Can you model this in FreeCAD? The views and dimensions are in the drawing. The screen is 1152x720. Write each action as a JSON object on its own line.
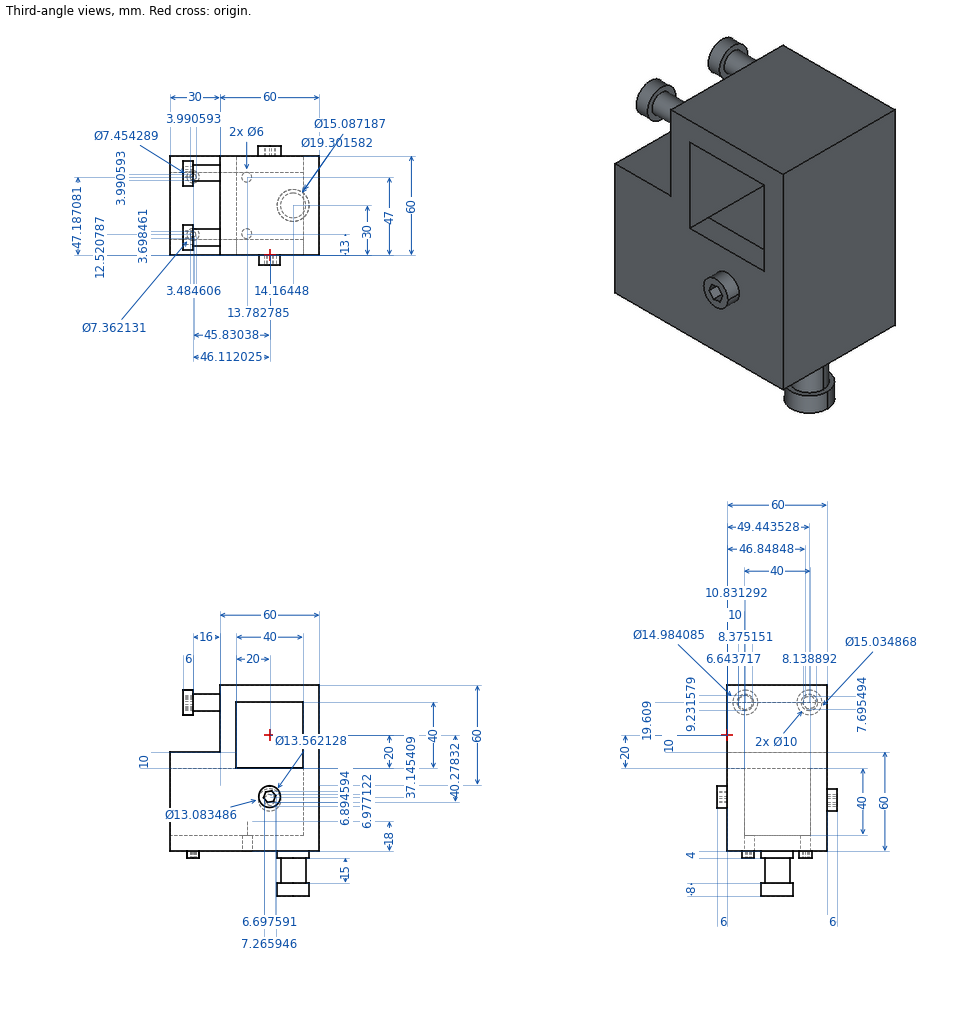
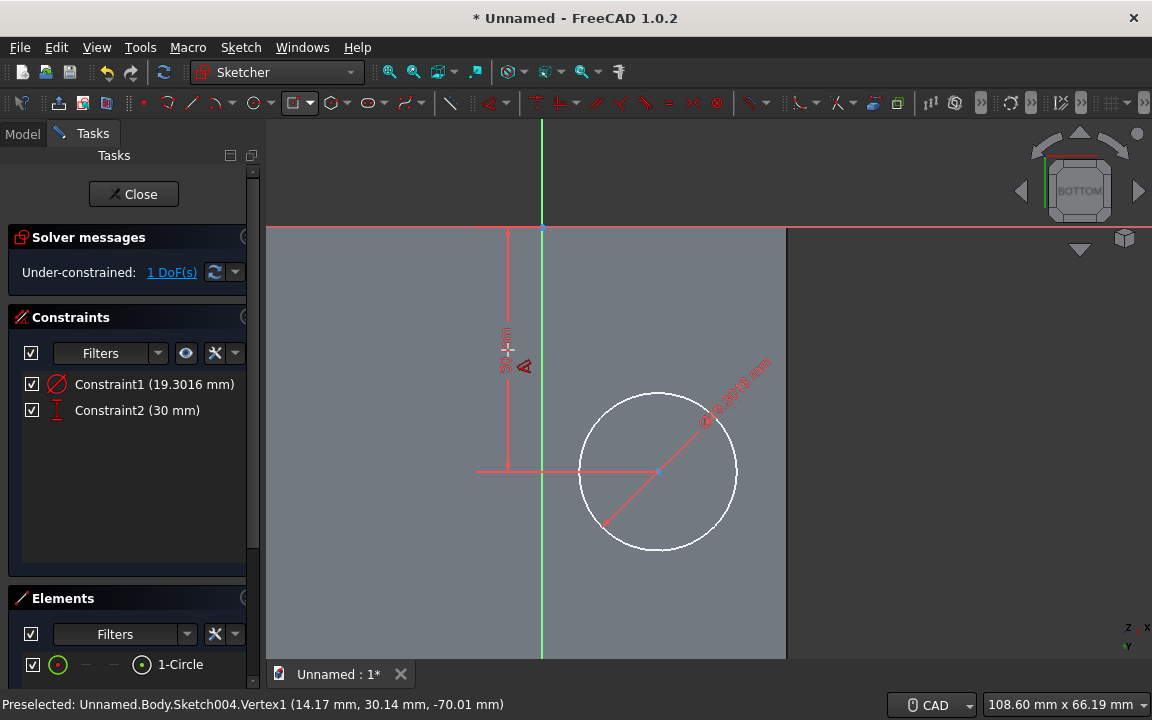
{"action": "left_click", "coordinate": [658, 472]}
{"action": "left_click", "coordinate": [600, 193]}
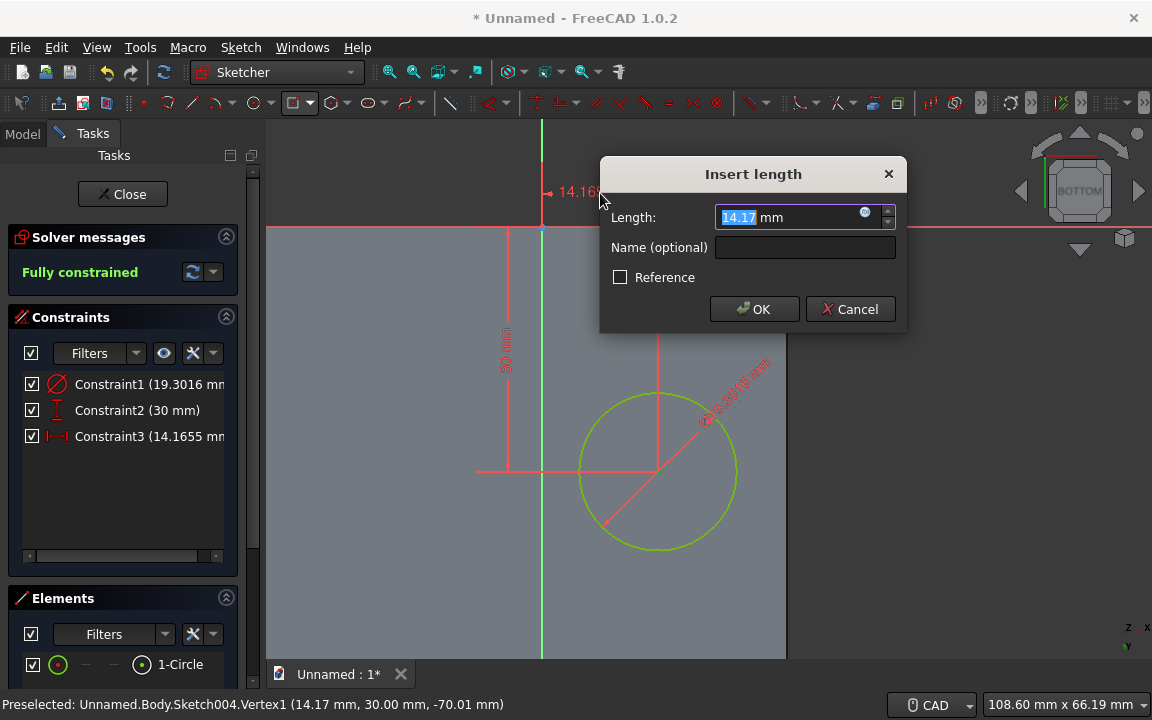
{"action": "type", "text": "14.16448"}
{"action": "key", "text": "Return"}
{"action": "key", "text": "Escape"}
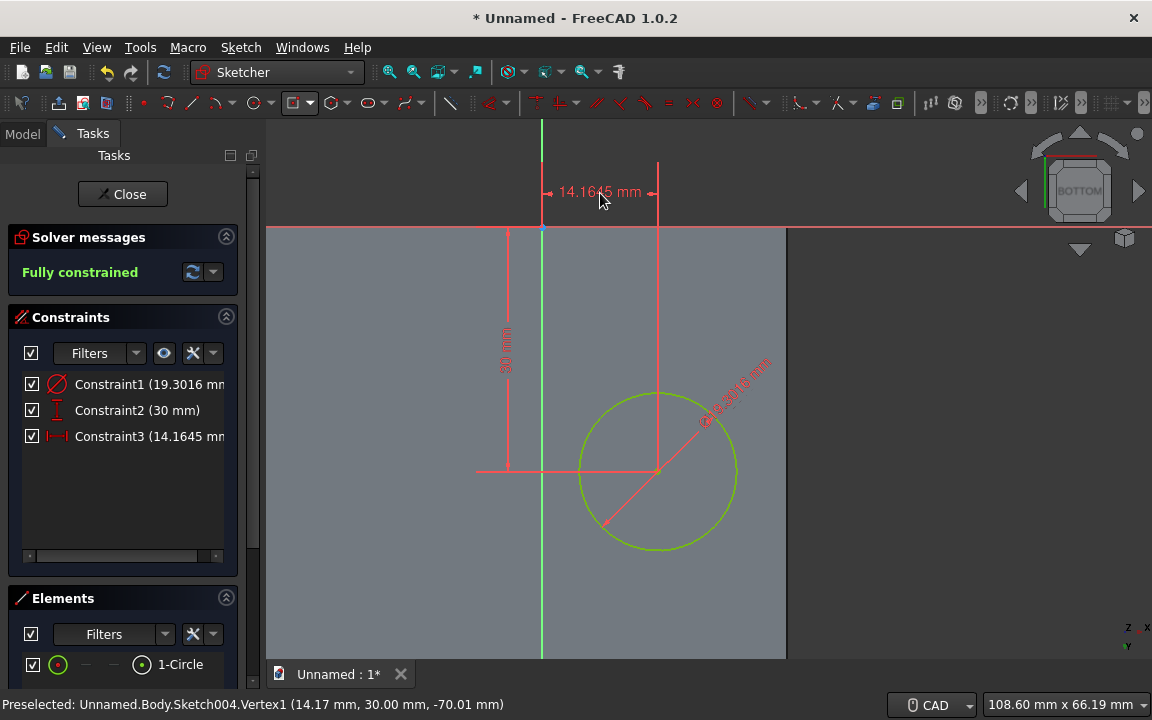
{"action": "left_click", "coordinate": [123, 194]}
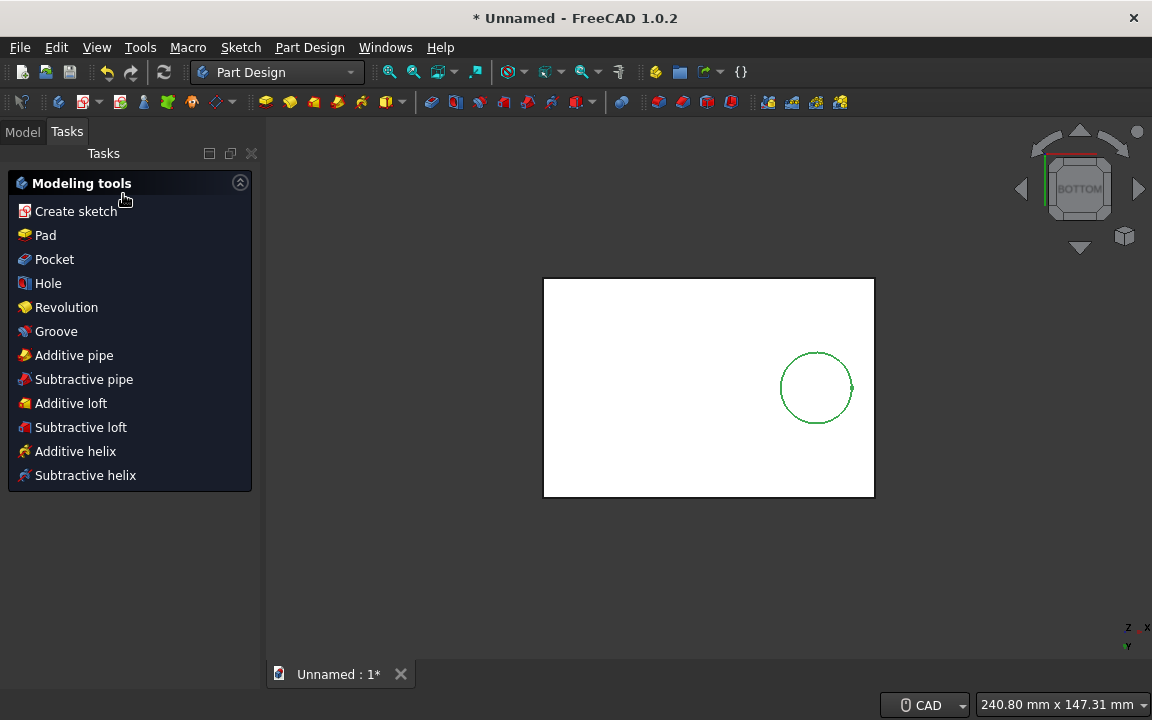
{"action": "left_click", "coordinate": [266, 102]}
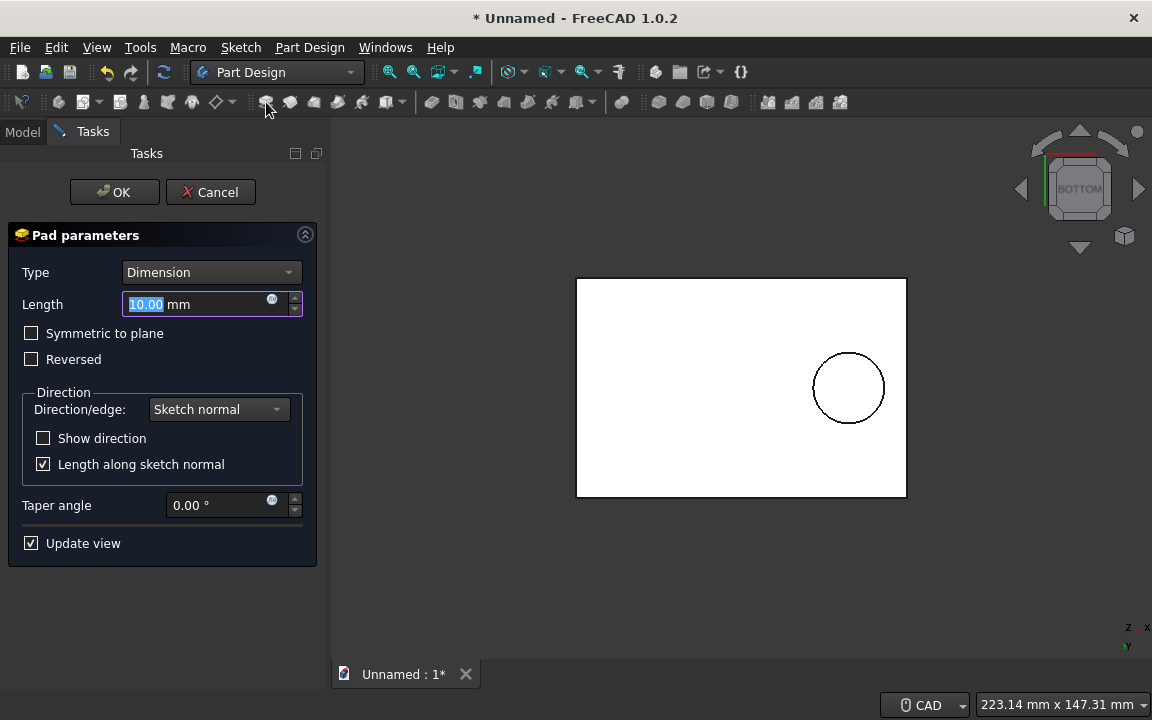
{"action": "type", "text": "4"}
{"action": "key", "text": "Tab"}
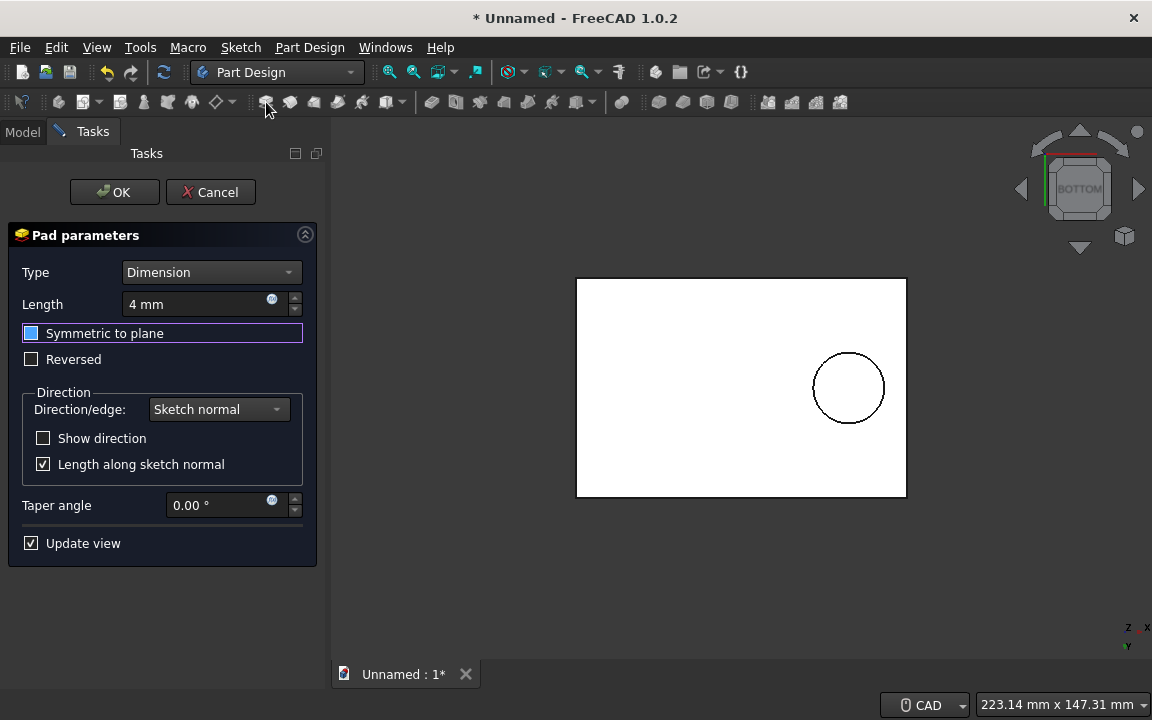
{"action": "left_click", "coordinate": [115, 192]}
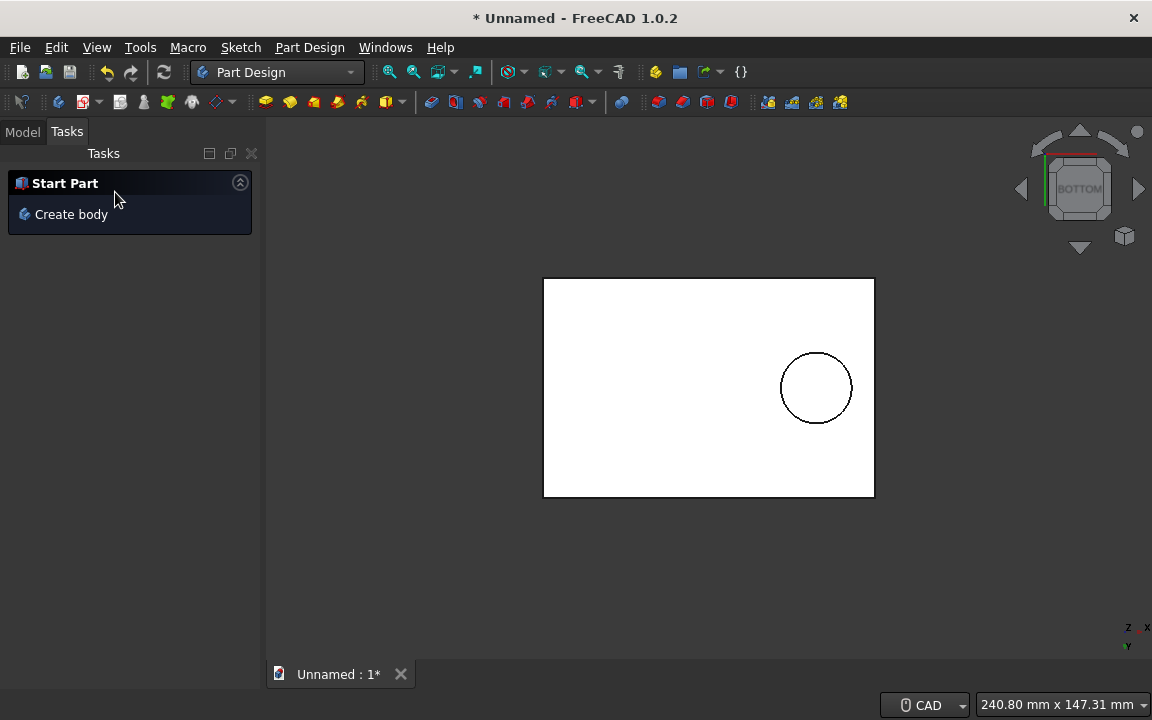
{"action": "left_click", "coordinate": [390, 72]}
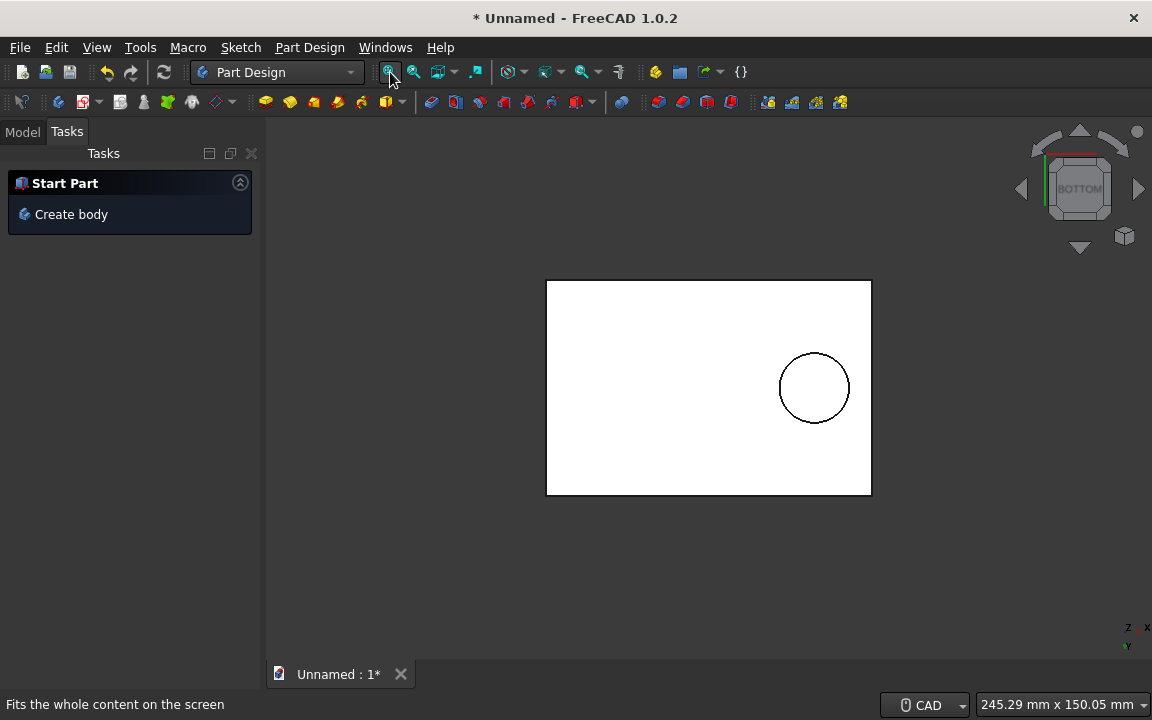
{"action": "left_click", "coordinate": [814, 387]}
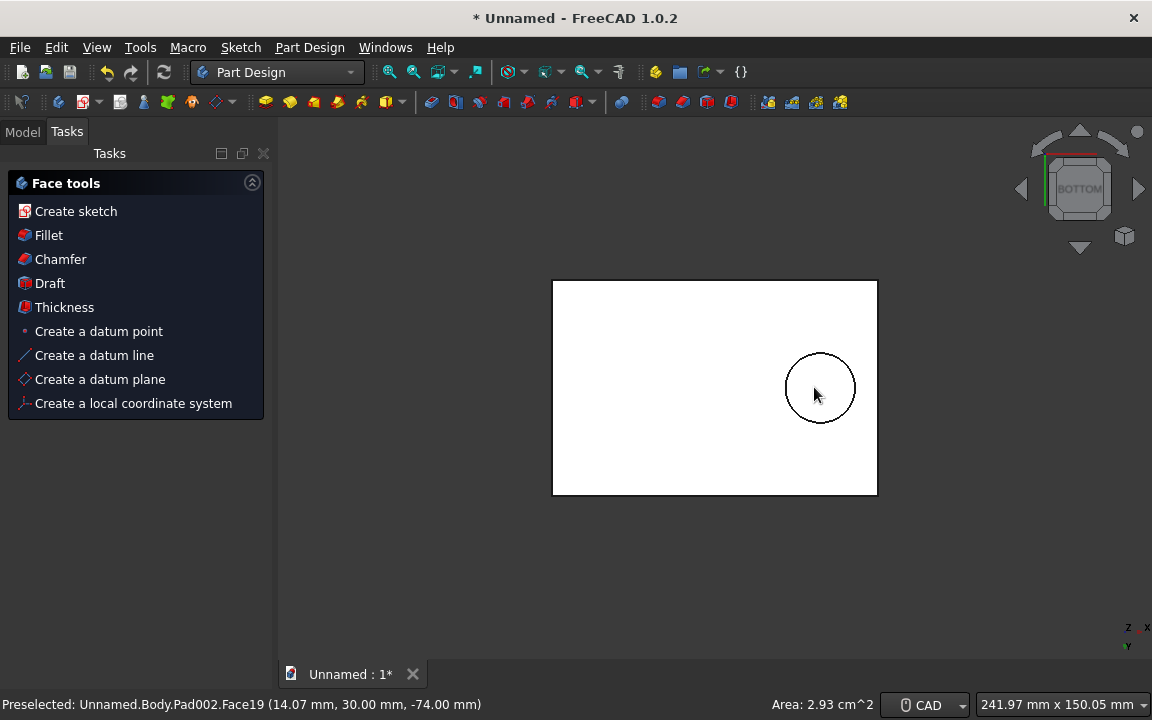
{"action": "left_click", "coordinate": [84, 102]}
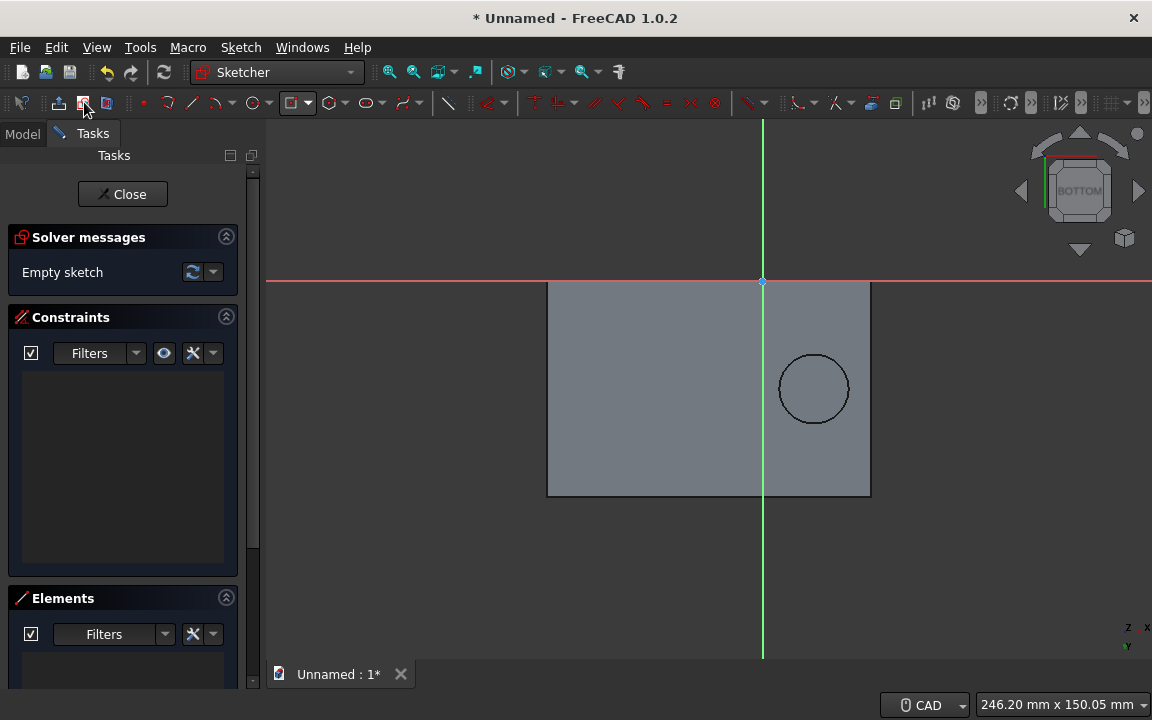
{"action": "scroll", "coordinate": [896, 325], "scroll_direction": "up", "scroll_amount": 5}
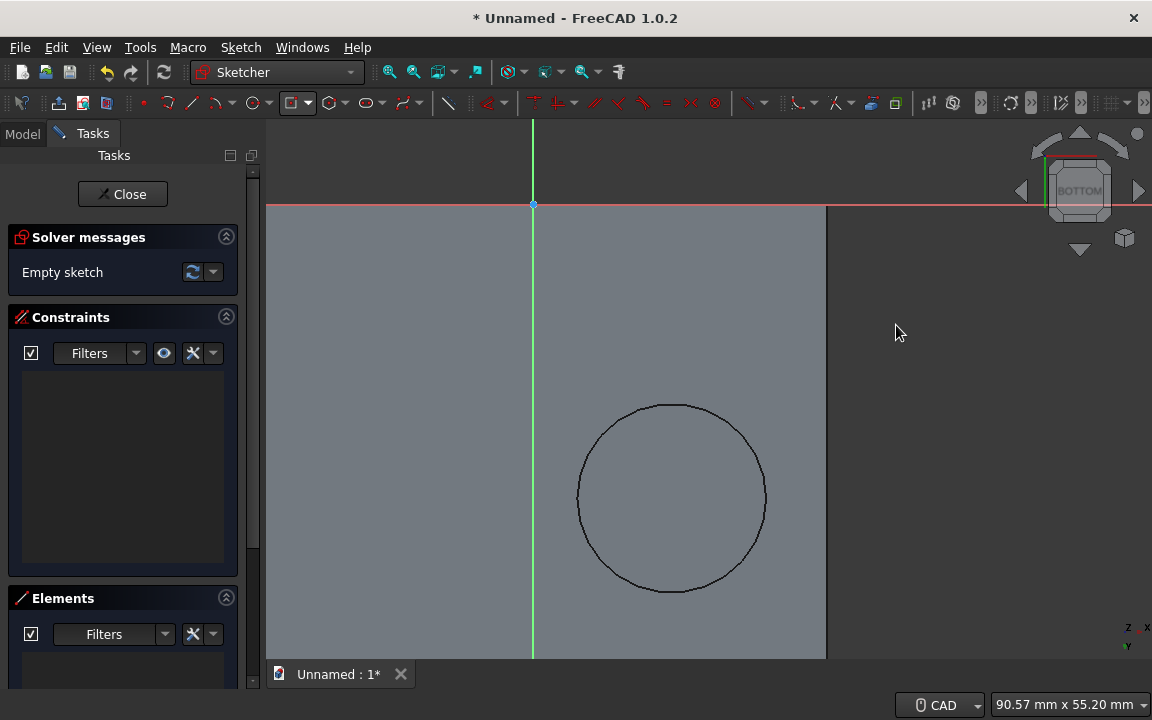
{"action": "left_click", "coordinate": [254, 104]}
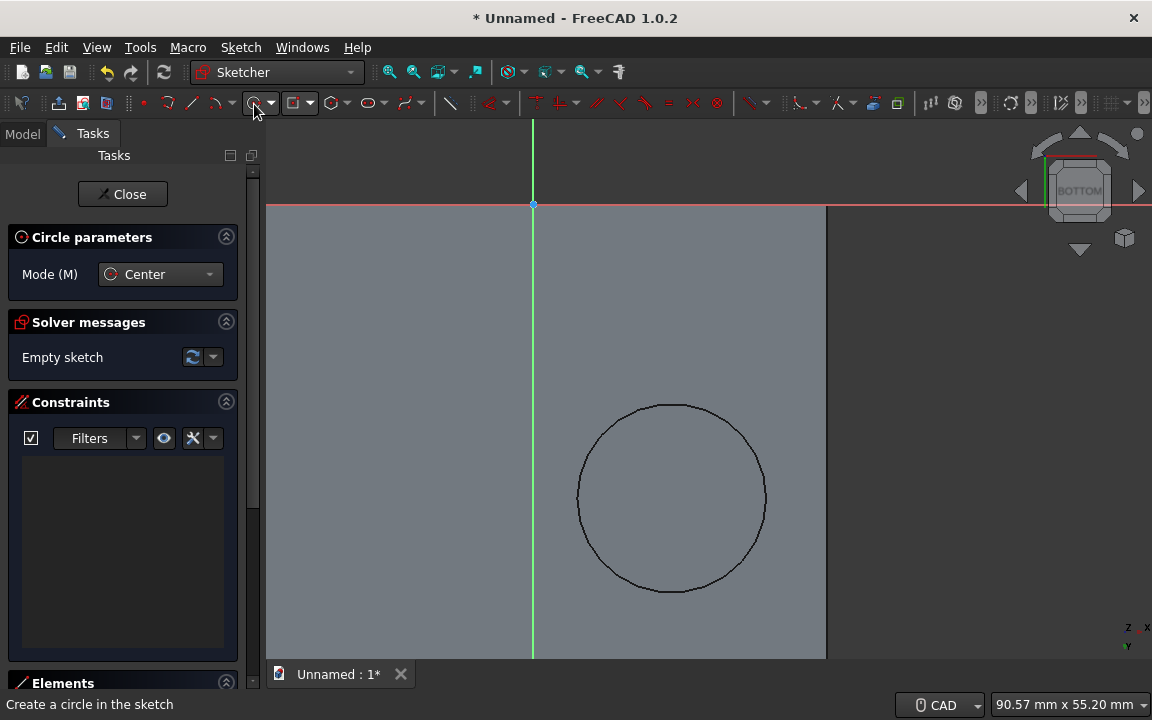
{"action": "left_click", "coordinate": [672, 498]}
{"action": "left_click", "coordinate": [724, 446]}
{"action": "key", "text": "Escape"}